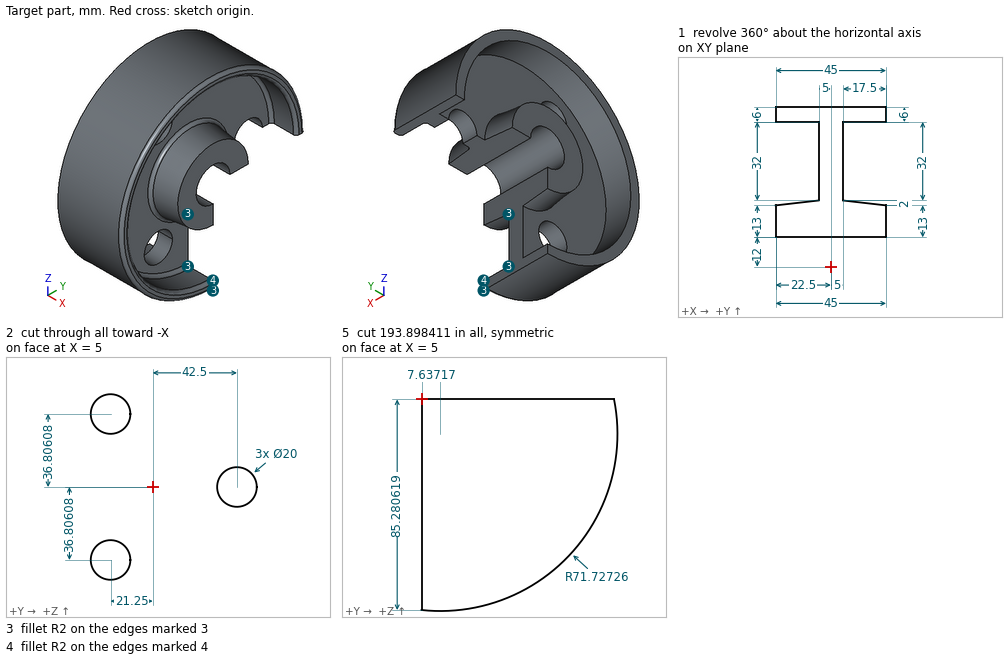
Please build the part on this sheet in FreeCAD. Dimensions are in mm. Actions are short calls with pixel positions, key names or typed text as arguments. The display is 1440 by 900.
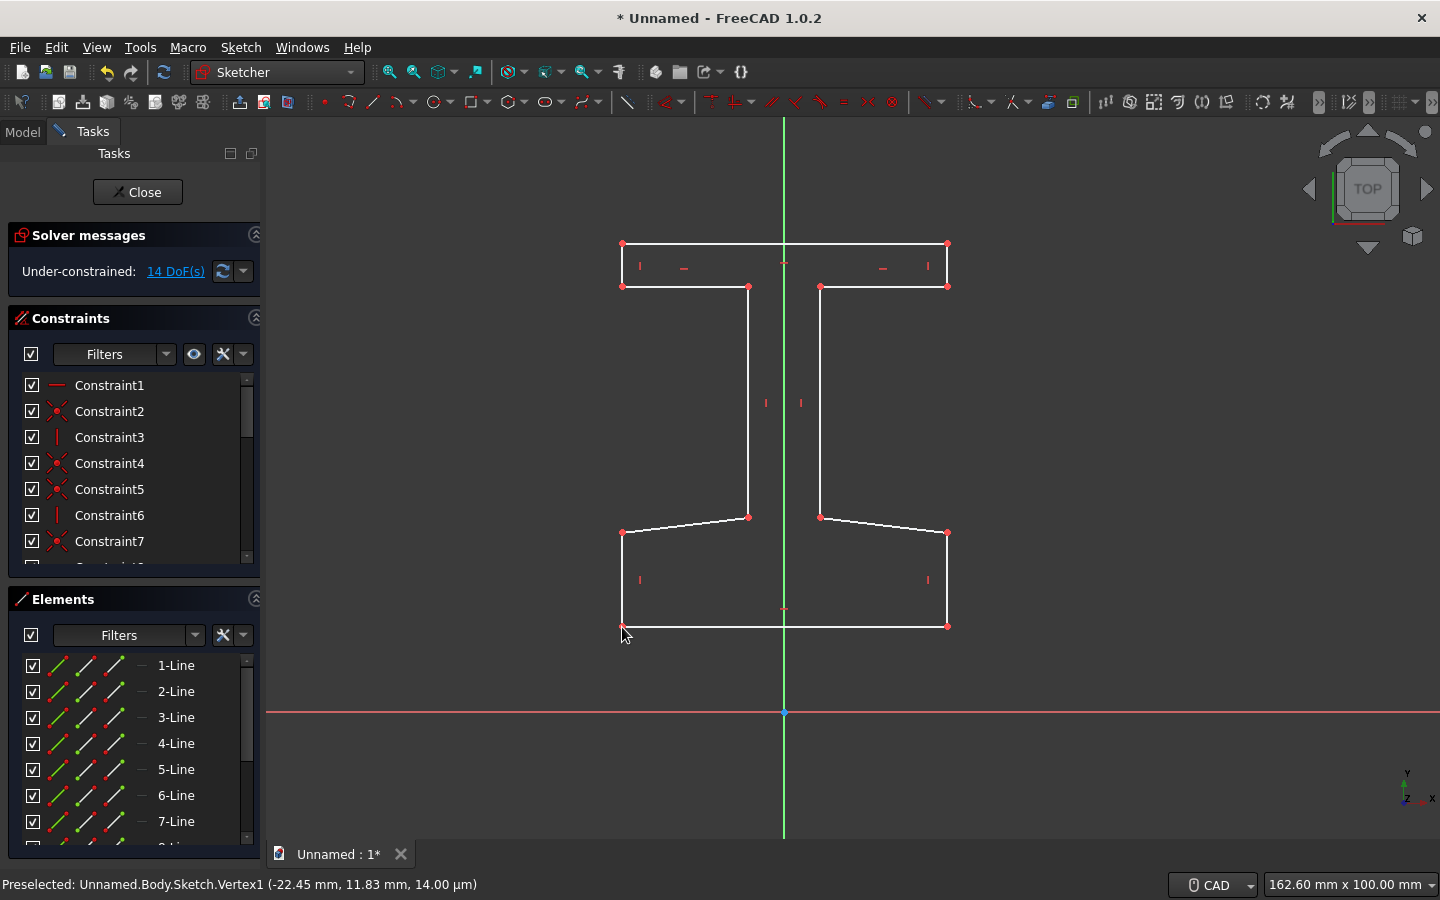
click(666, 102)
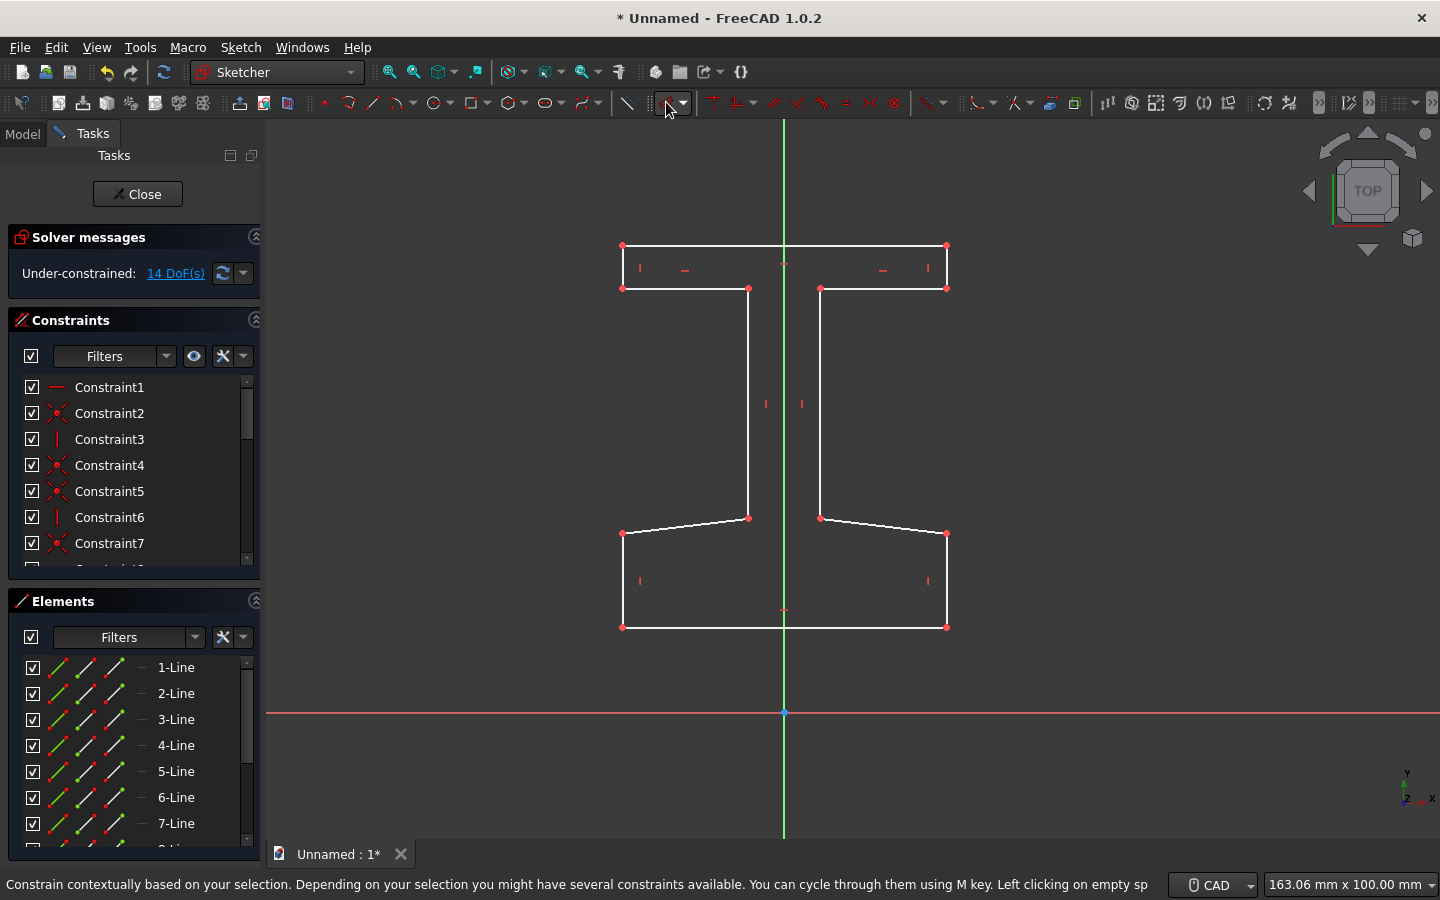
click(947, 276)
click(981, 267)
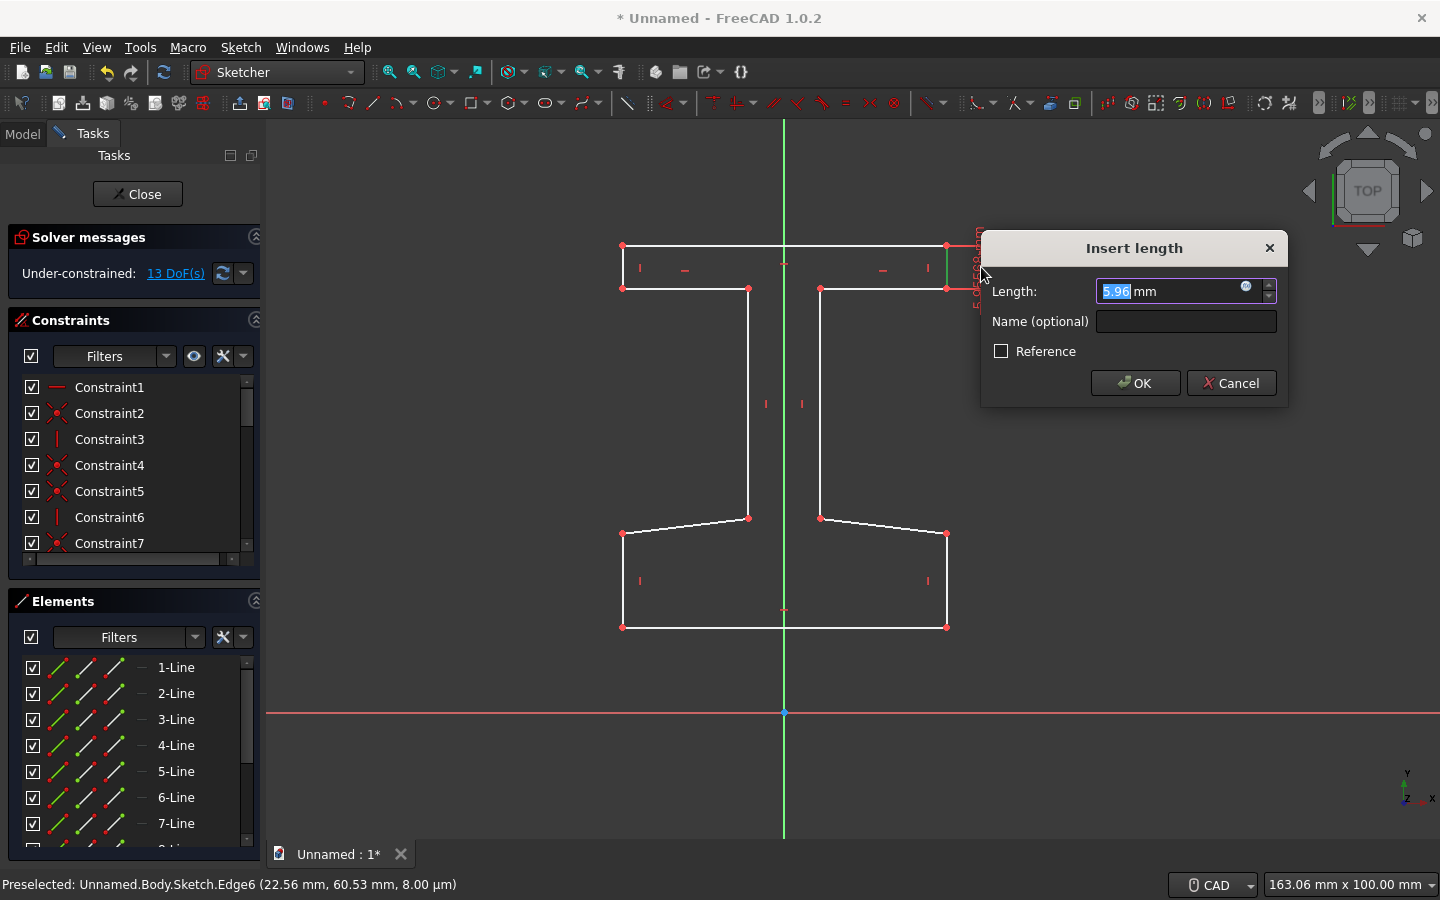
text(6)
key(Return)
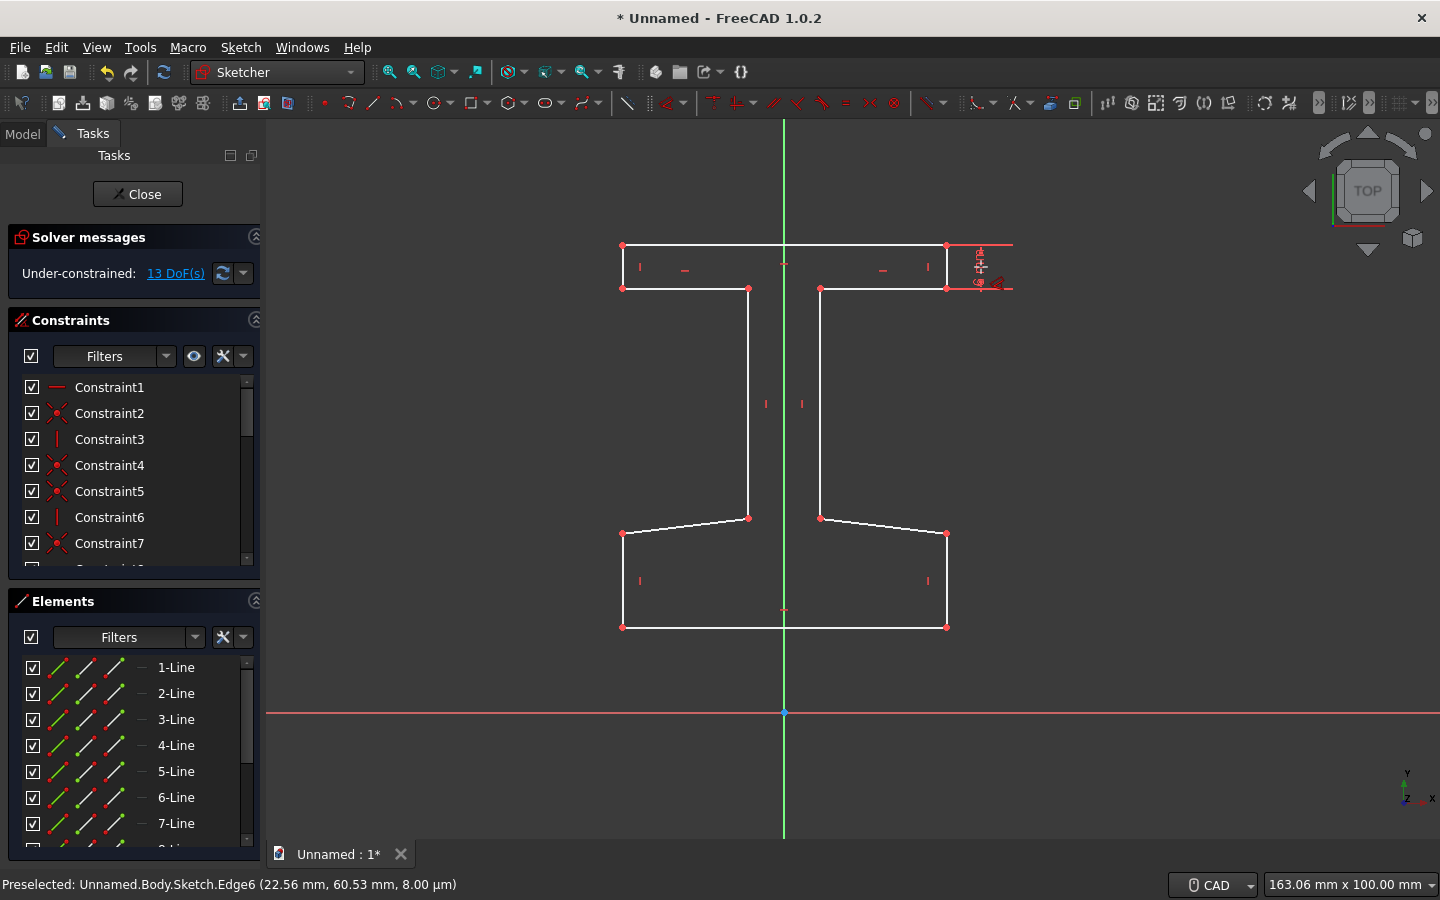
click(623, 258)
click(589, 267)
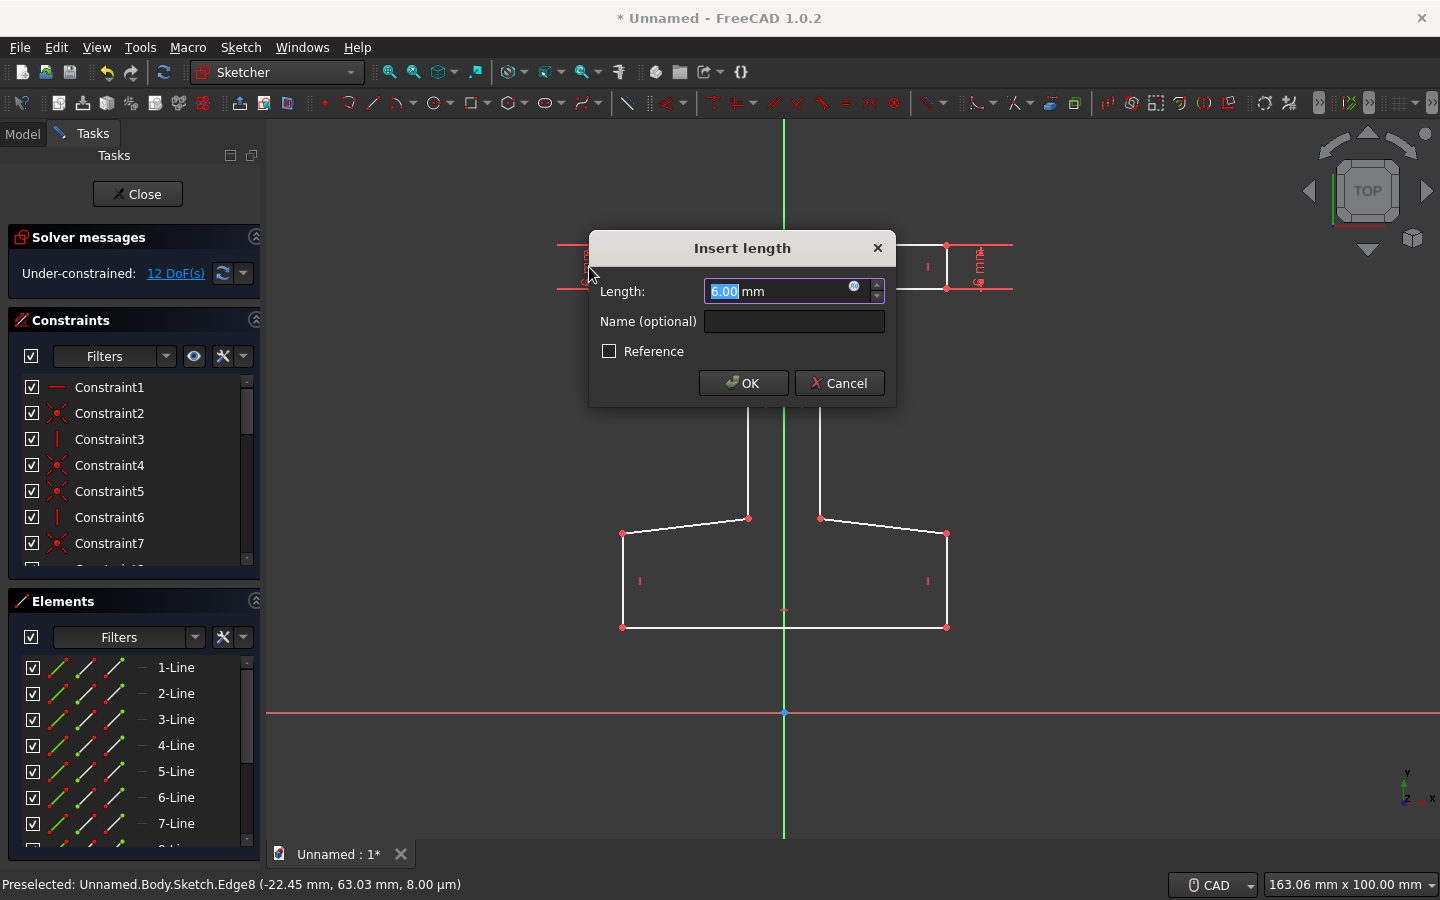
text(6)
key(Return)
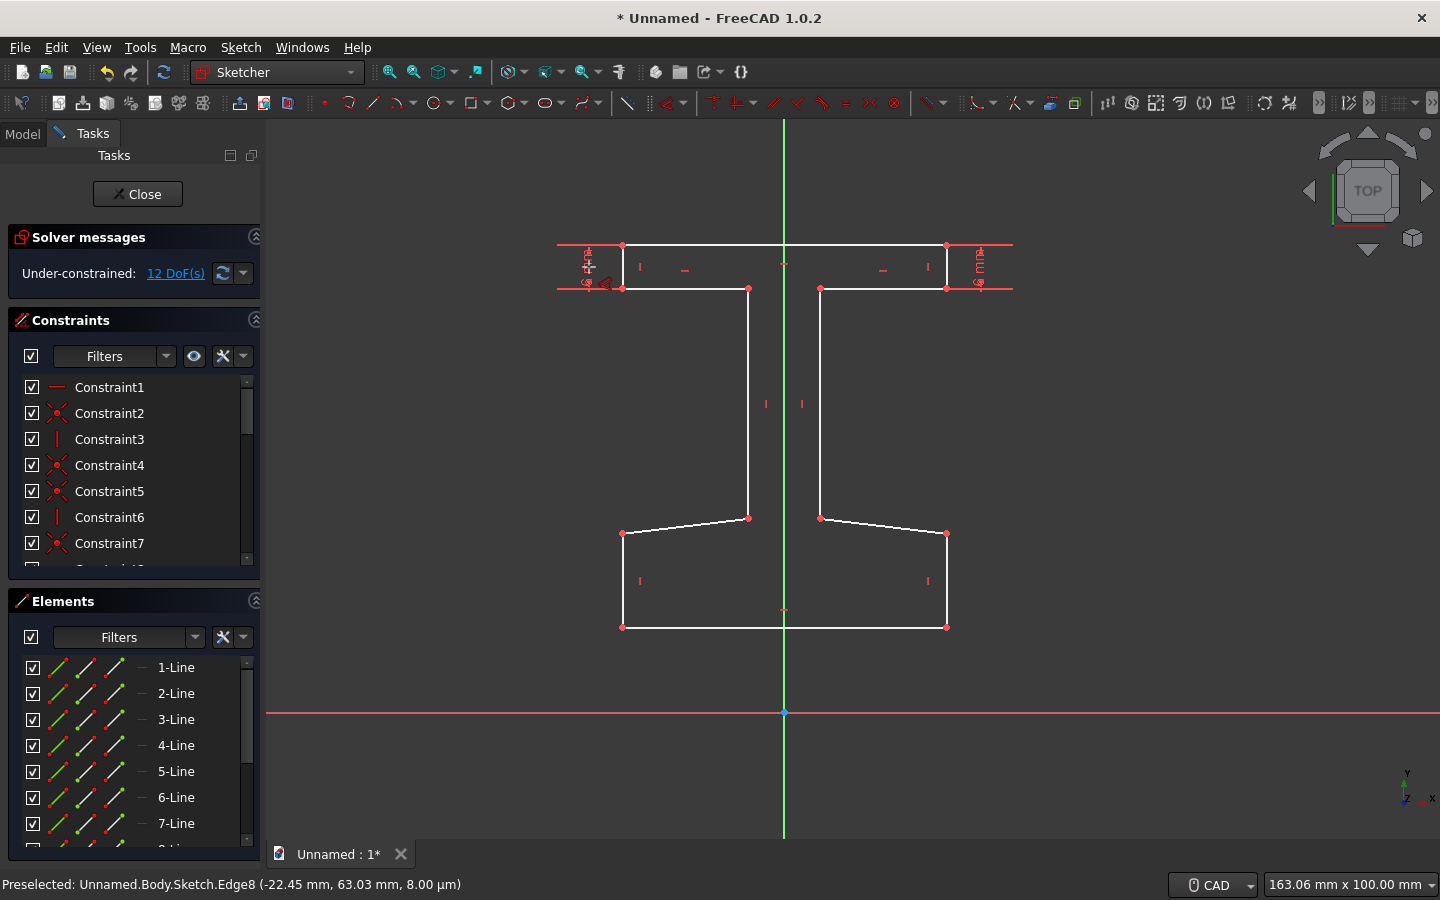
click(720, 628)
click(710, 662)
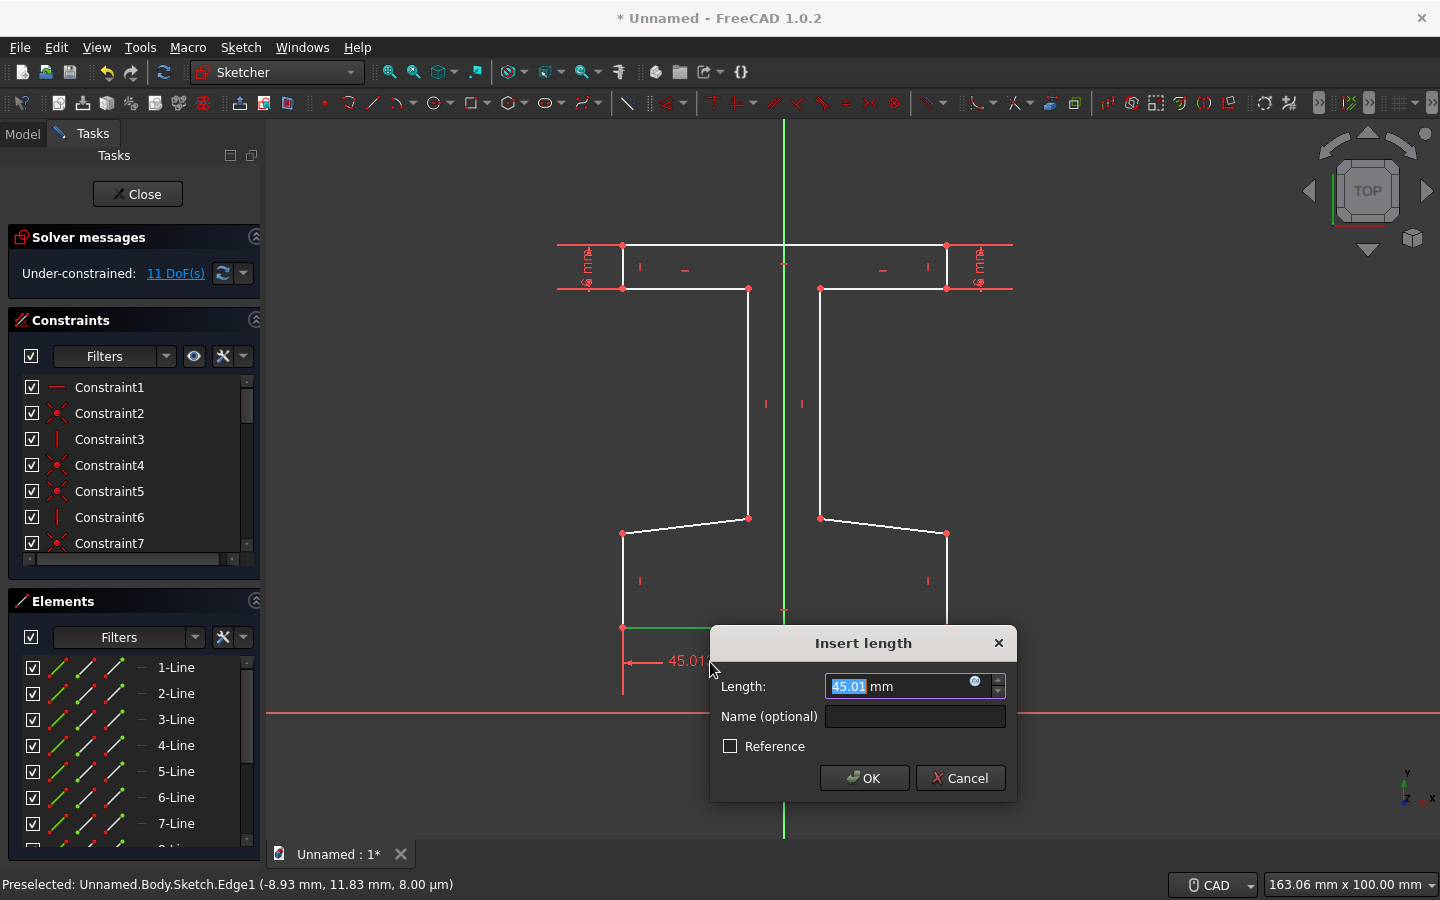
text(45)
key(Return)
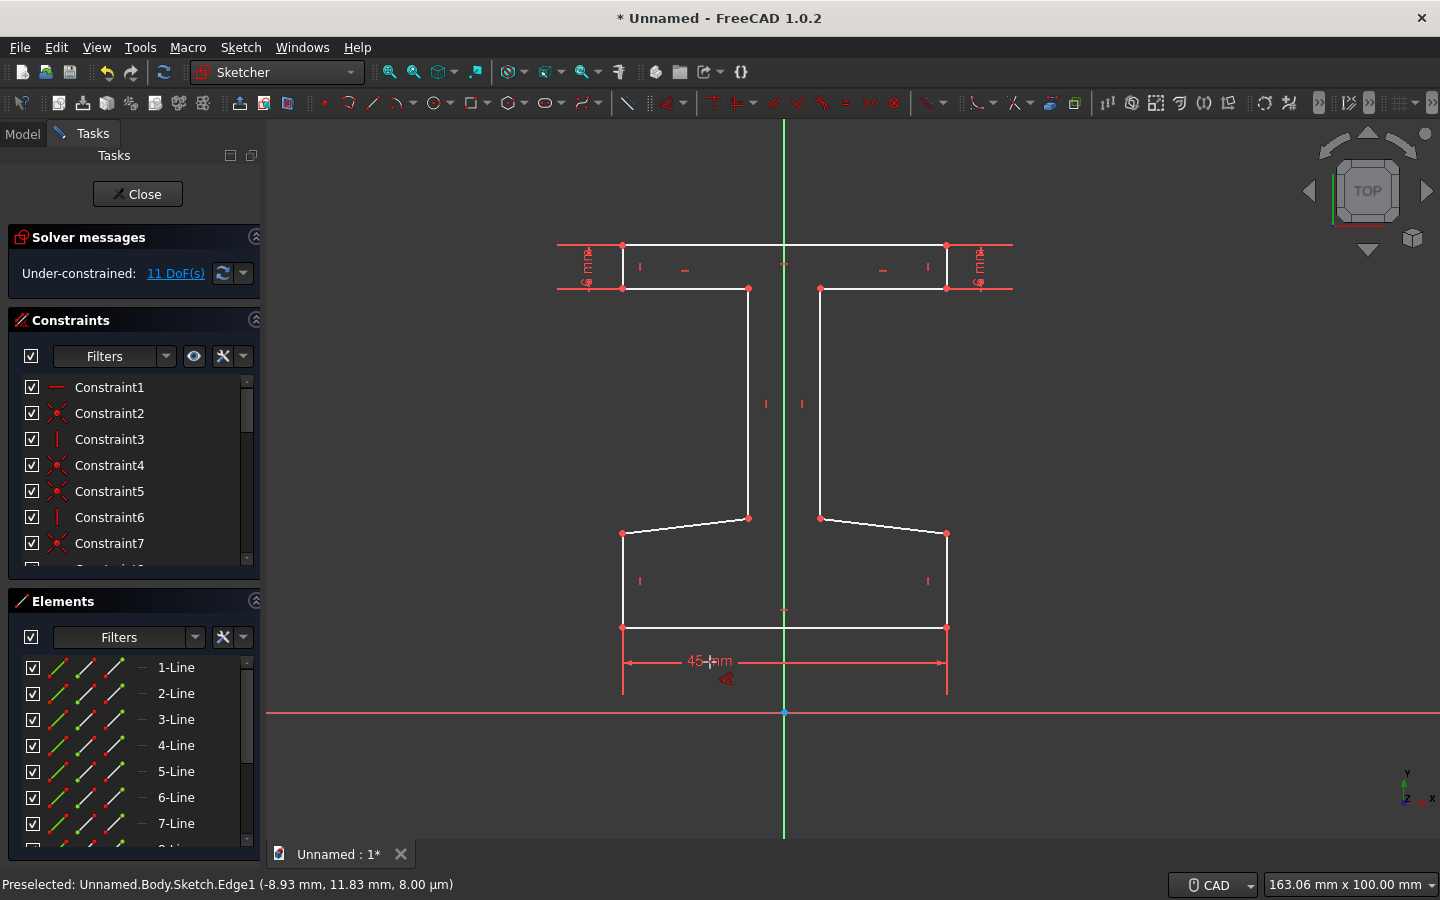
click(947, 599)
click(981, 581)